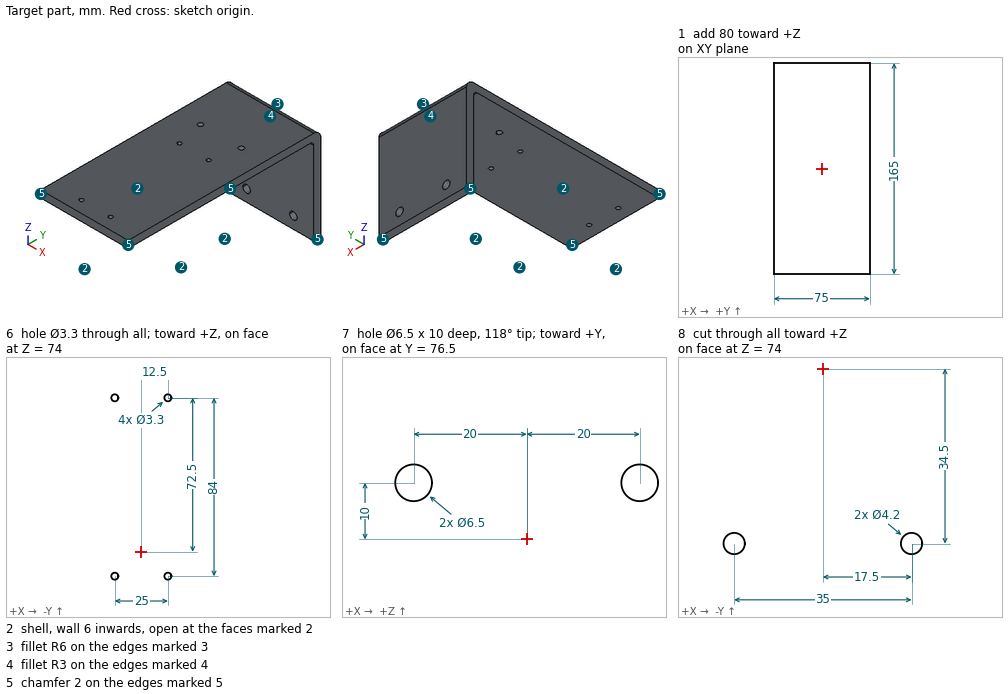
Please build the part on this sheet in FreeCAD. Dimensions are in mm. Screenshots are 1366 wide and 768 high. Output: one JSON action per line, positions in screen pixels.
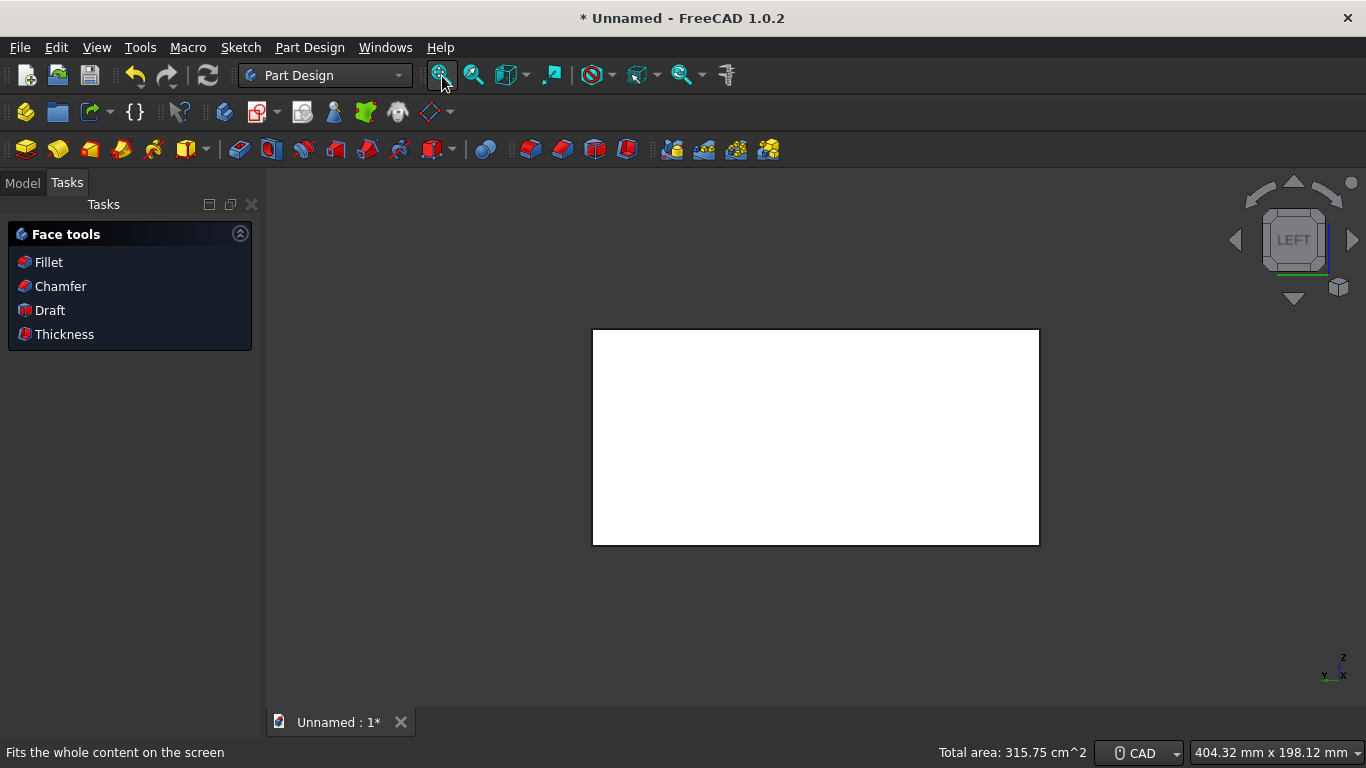
{"action": "left_click", "coordinate": [442, 76]}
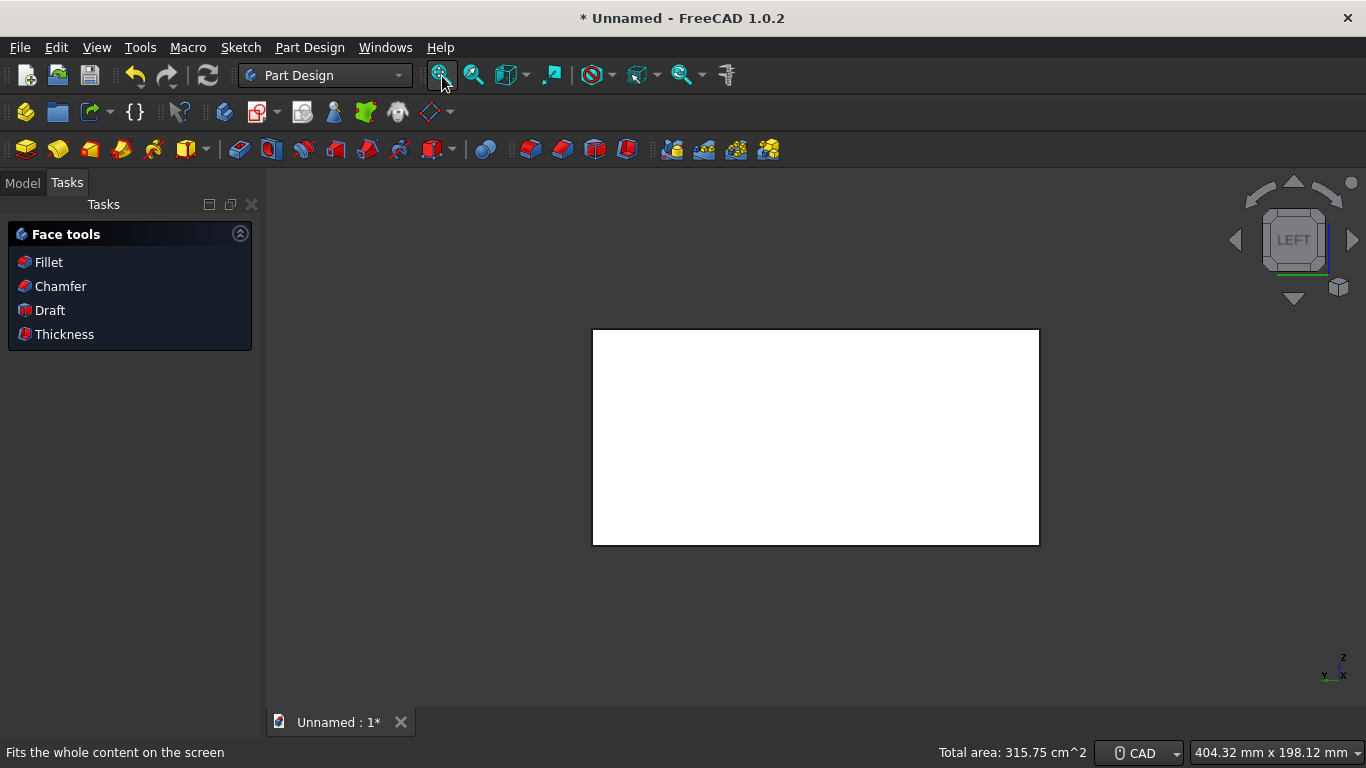
{"action": "left_click", "coordinate": [752, 436], "text": "ctrl"}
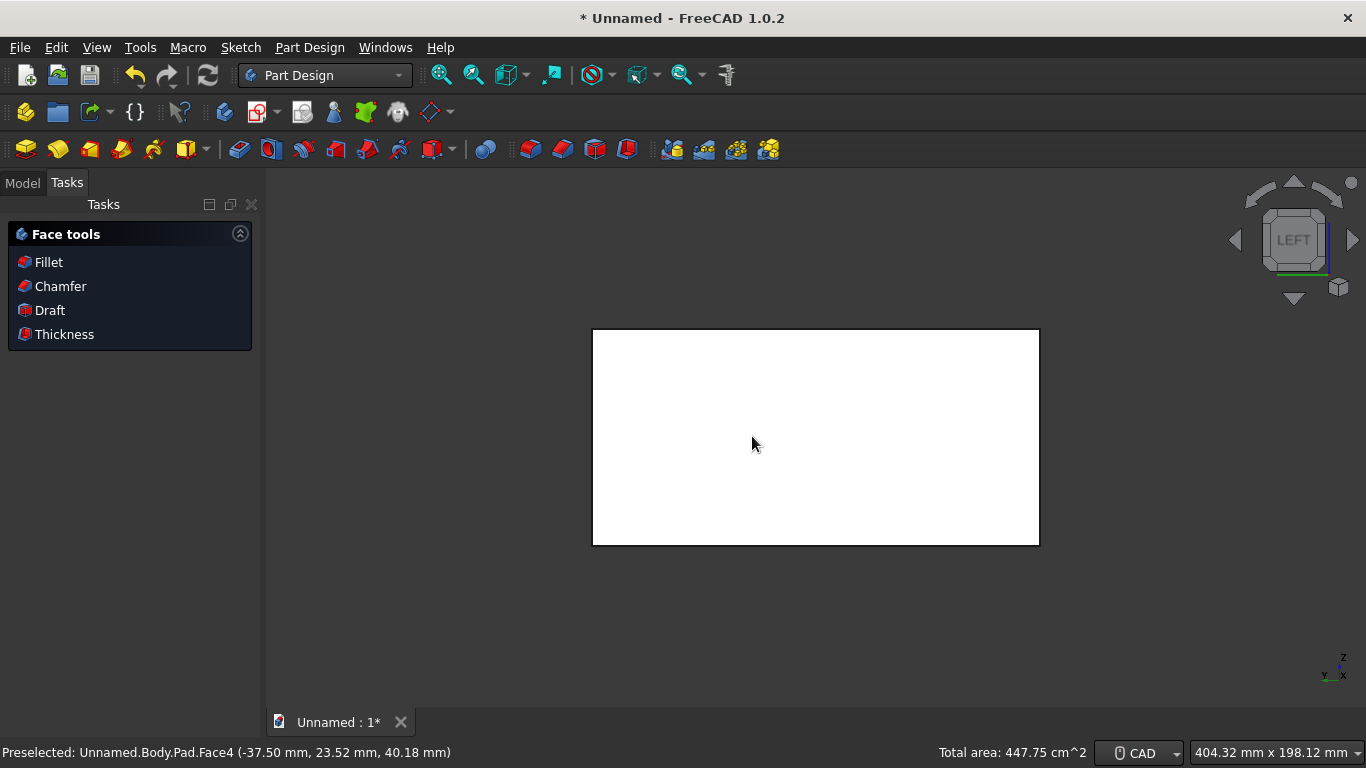
{"action": "left_click", "coordinate": [628, 150]}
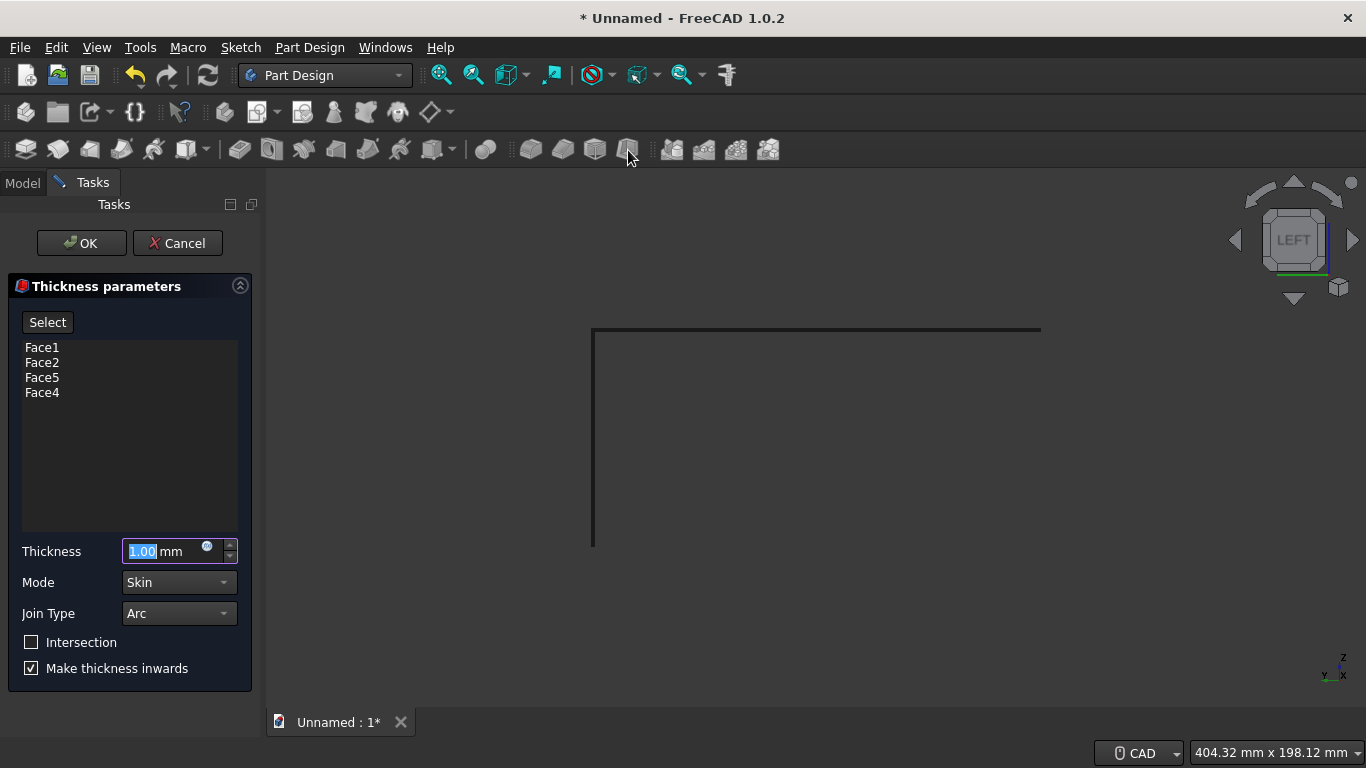
{"action": "type", "text": "6"}
{"action": "key", "text": "Tab"}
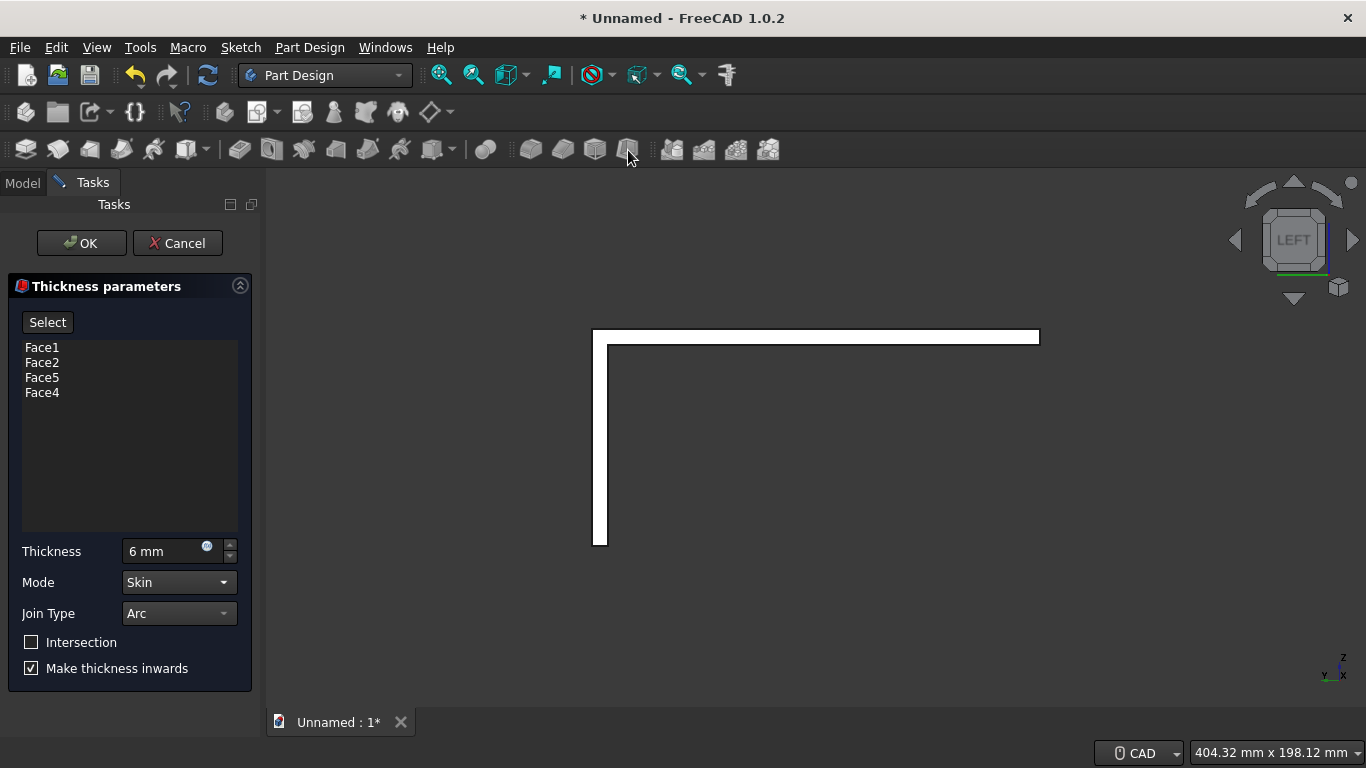
{"action": "left_click", "coordinate": [180, 614]}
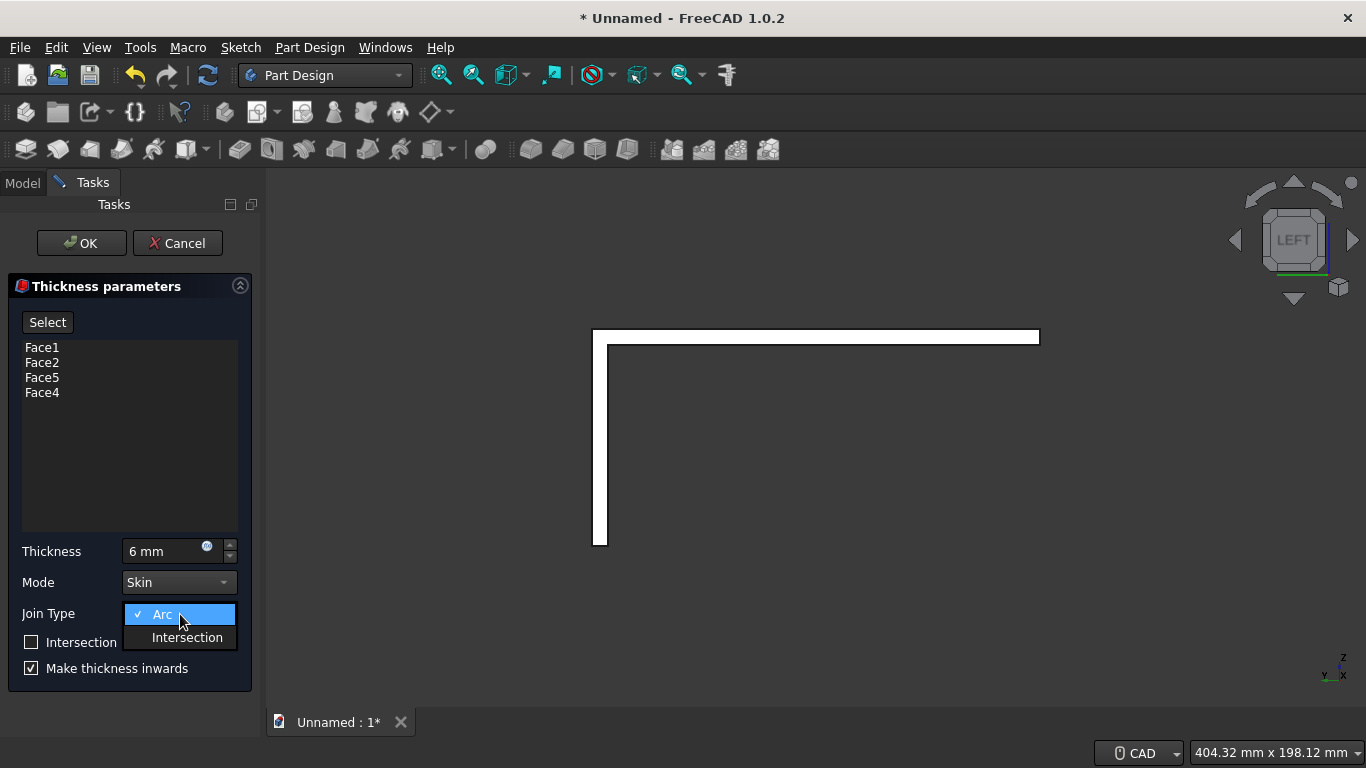
{"action": "left_click", "coordinate": [179, 638]}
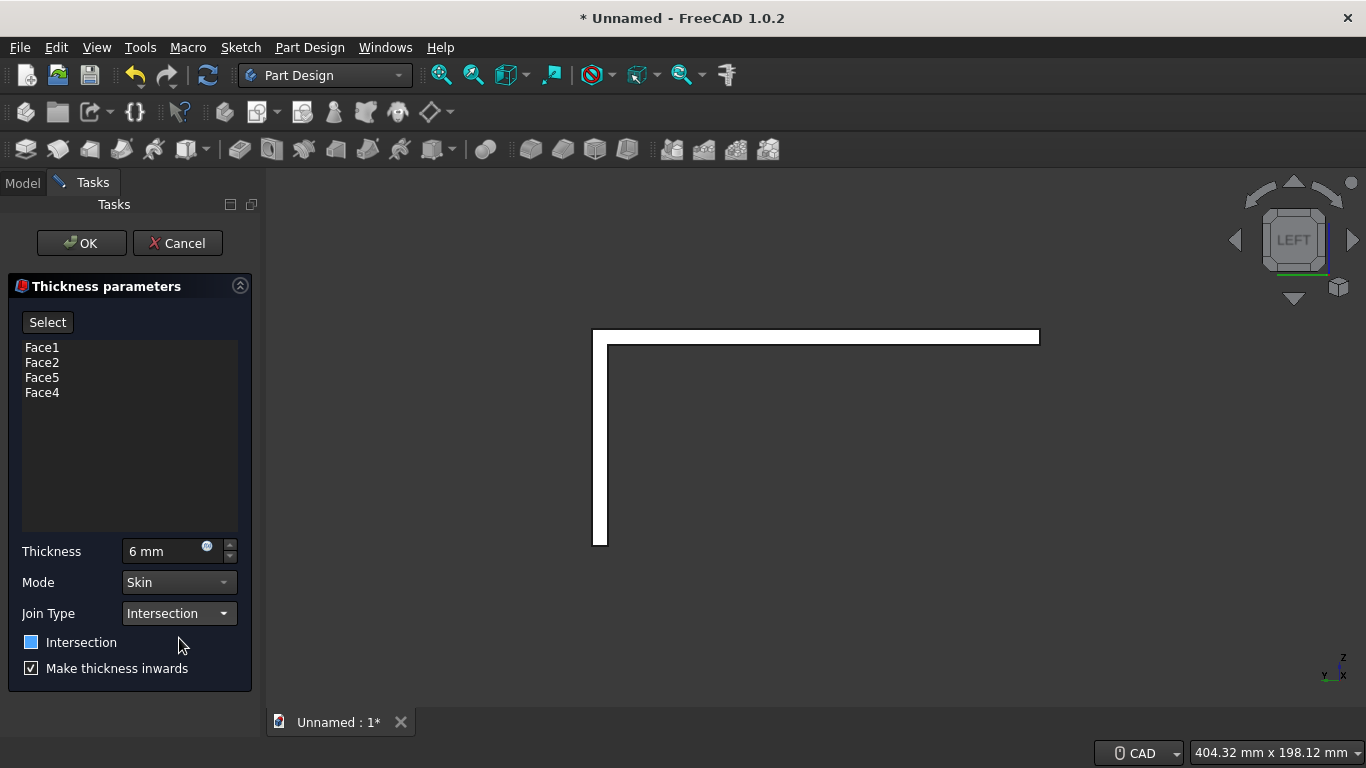
{"action": "left_click", "coordinate": [82, 243]}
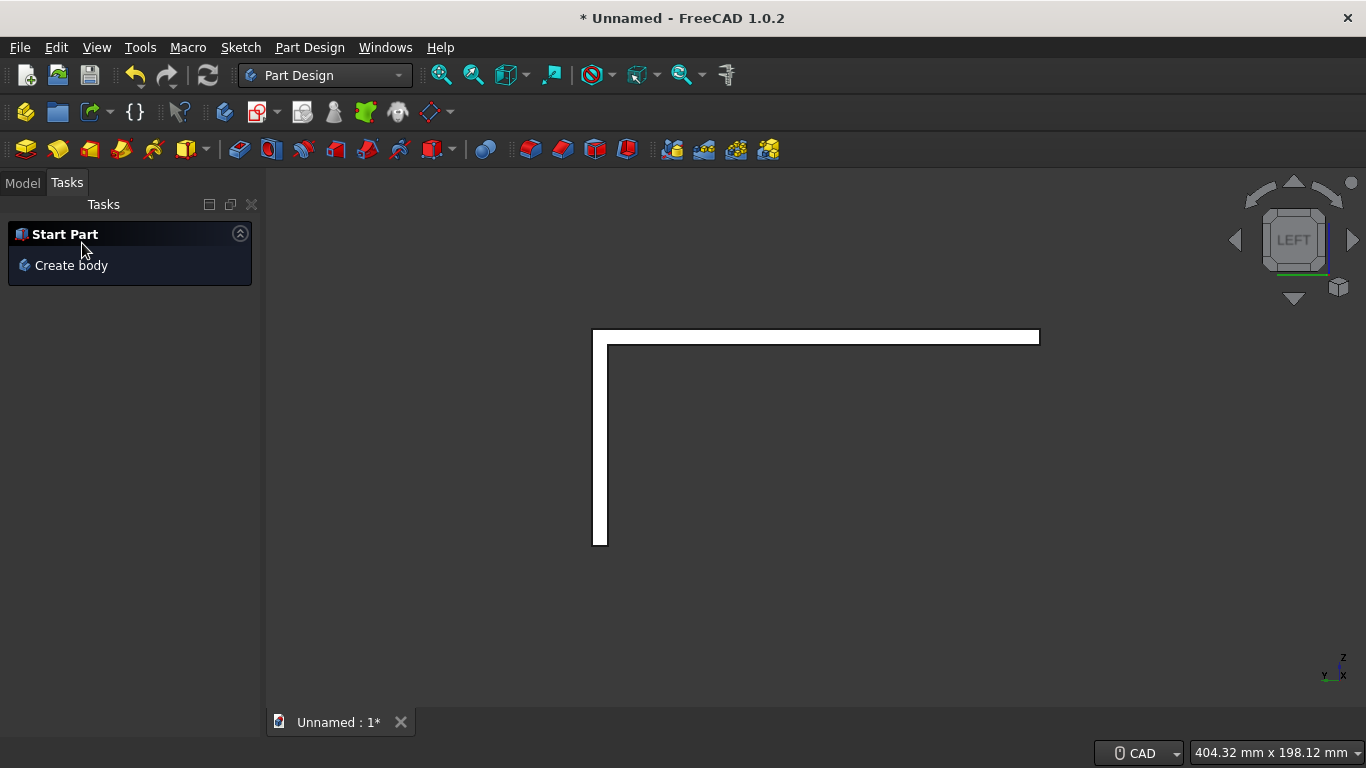
{"action": "left_click", "coordinate": [442, 76]}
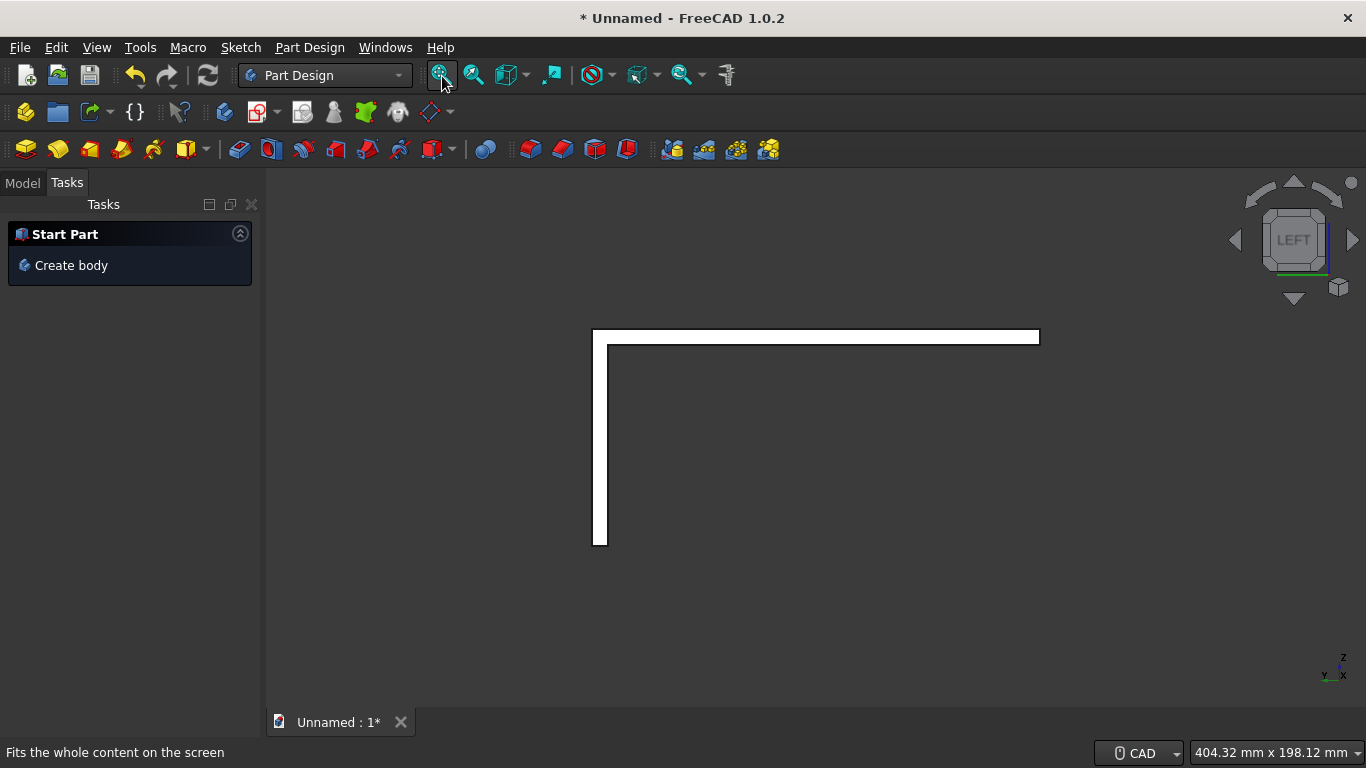
{"action": "key", "text": "0"}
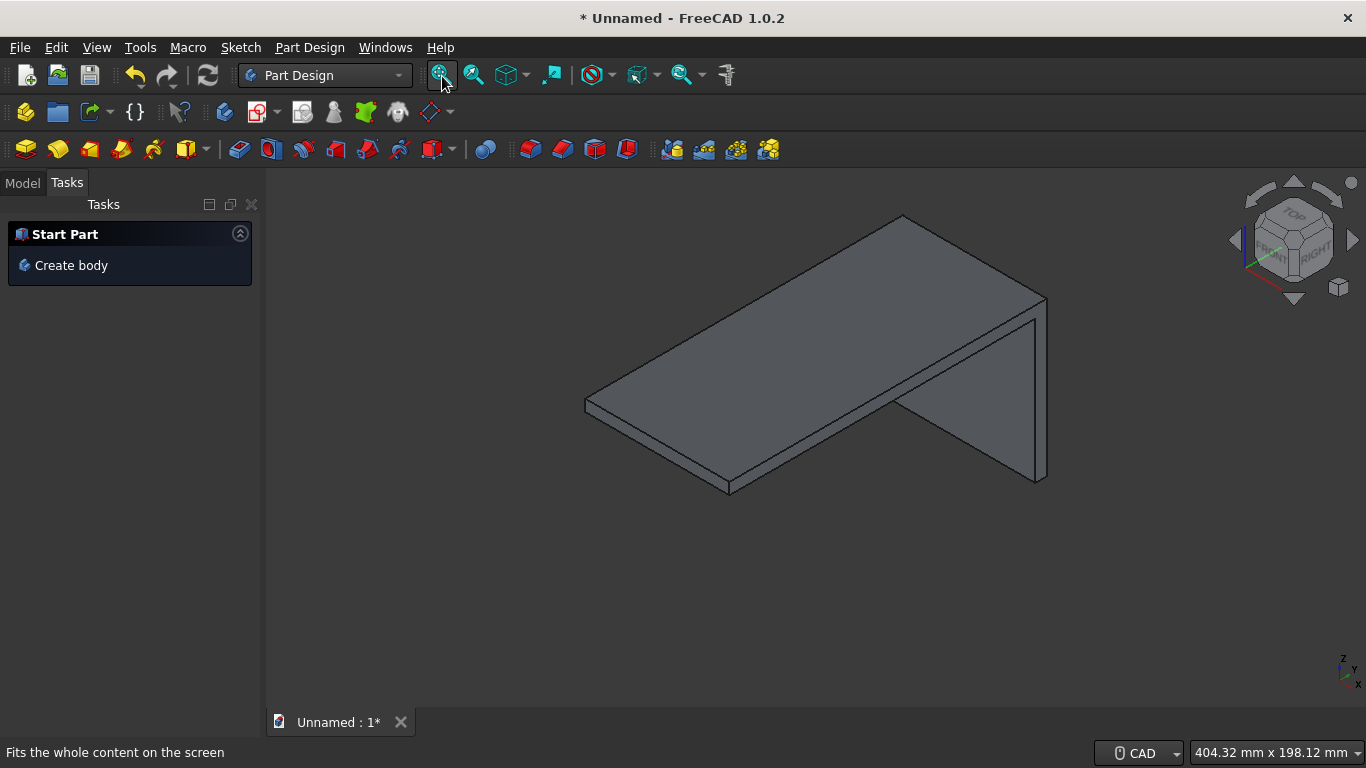
{"action": "key", "text": "2"}